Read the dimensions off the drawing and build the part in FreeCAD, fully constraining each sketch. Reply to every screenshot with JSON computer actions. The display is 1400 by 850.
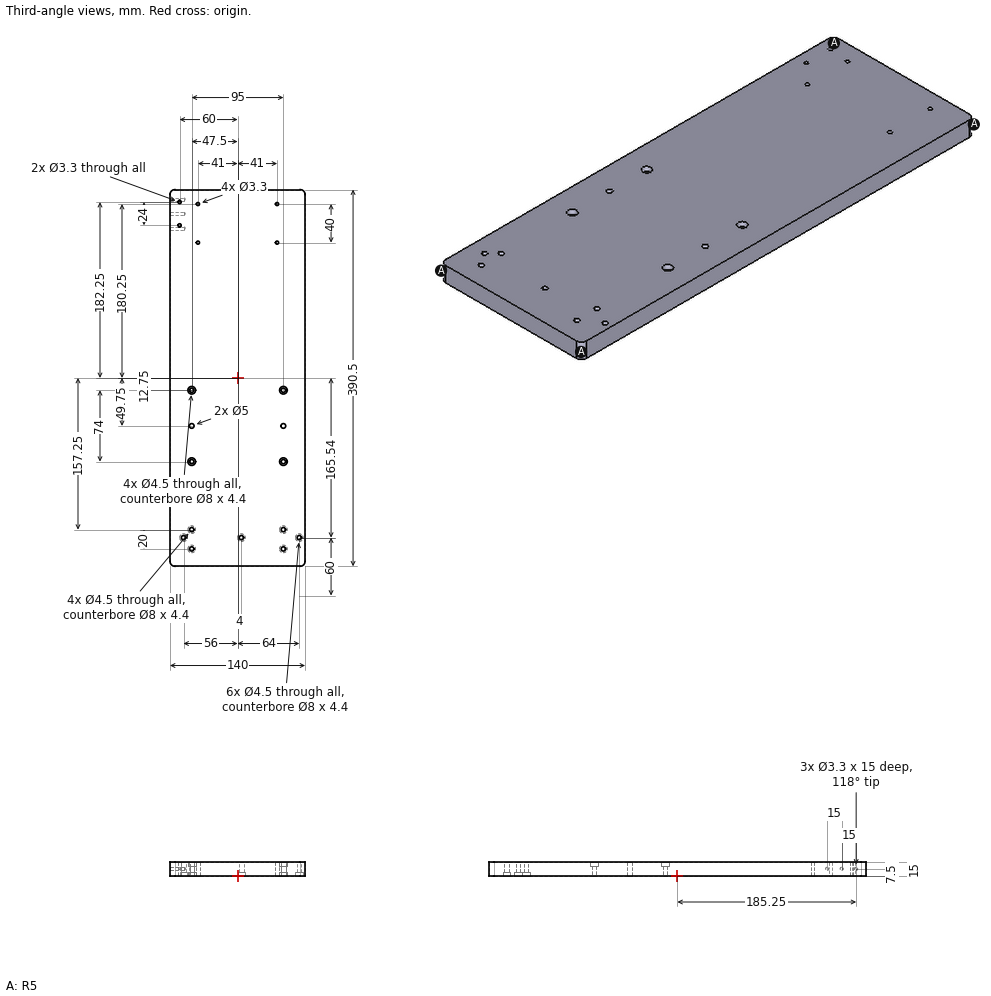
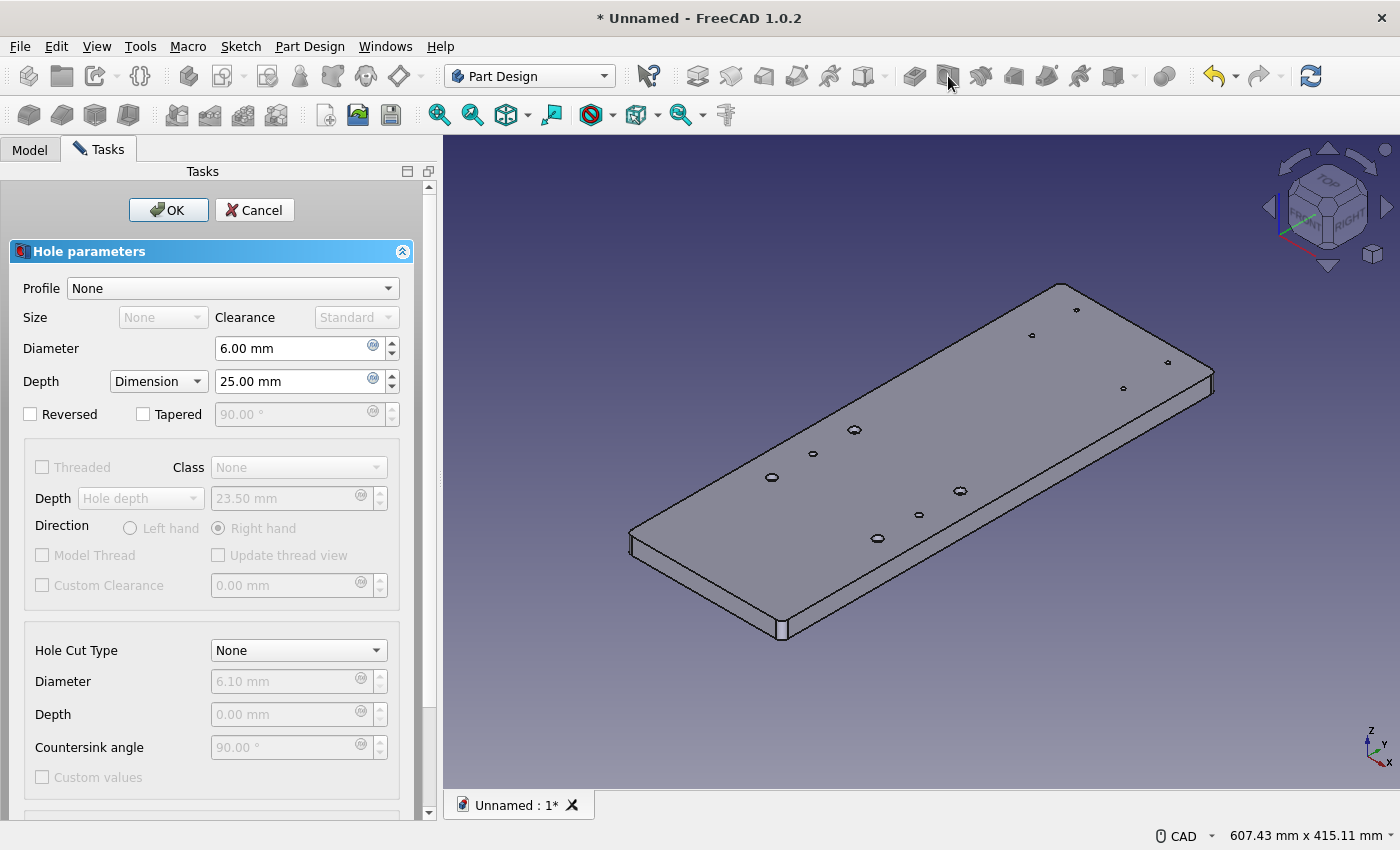
{"action": "triple_click", "coordinate": [300, 348]}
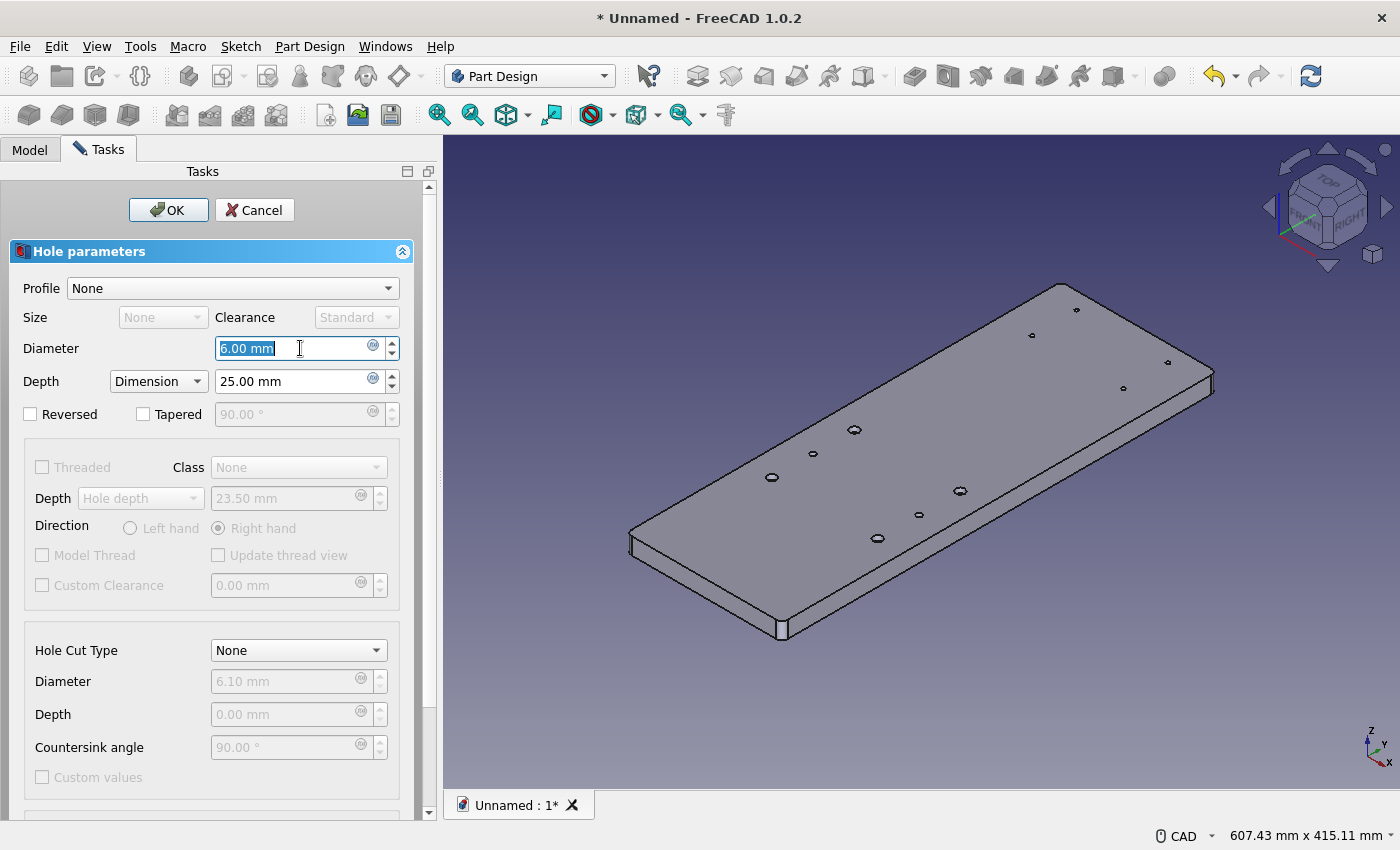
{"action": "type", "text": "4.5"}
{"action": "key", "text": "Tab"}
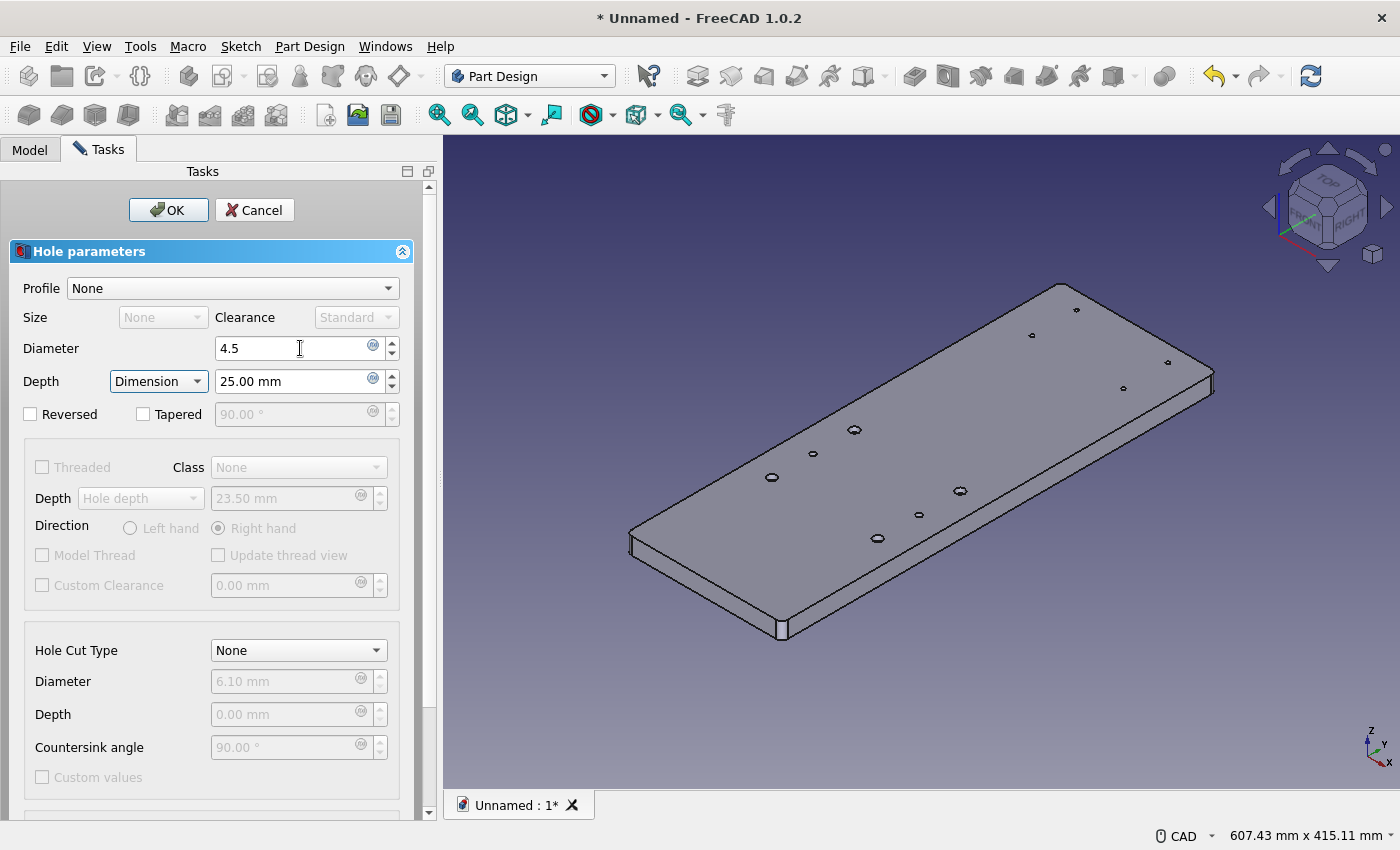
{"action": "left_click", "coordinate": [160, 382]}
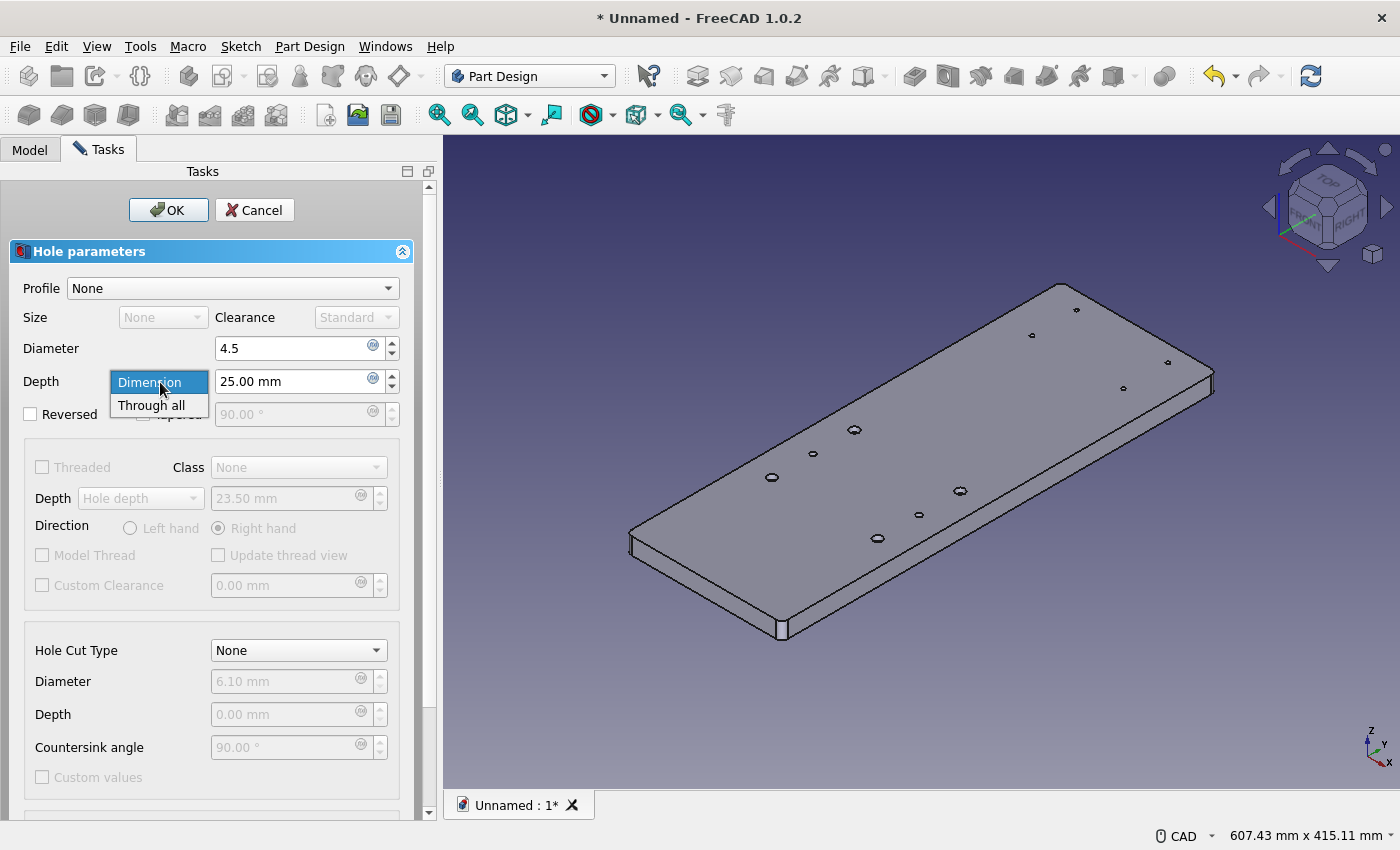
{"action": "left_click", "coordinate": [158, 406]}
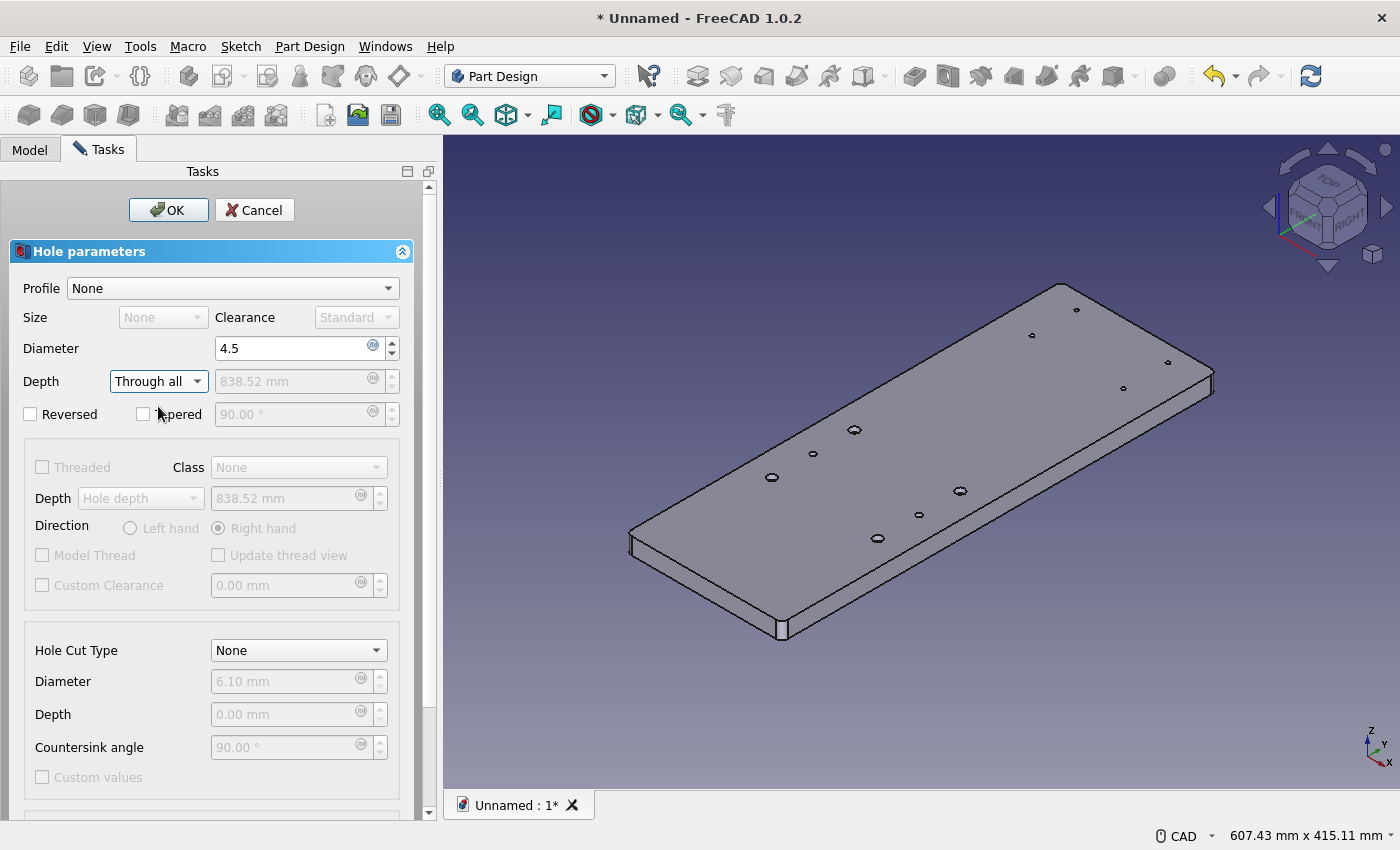
{"action": "left_click", "coordinate": [31, 414]}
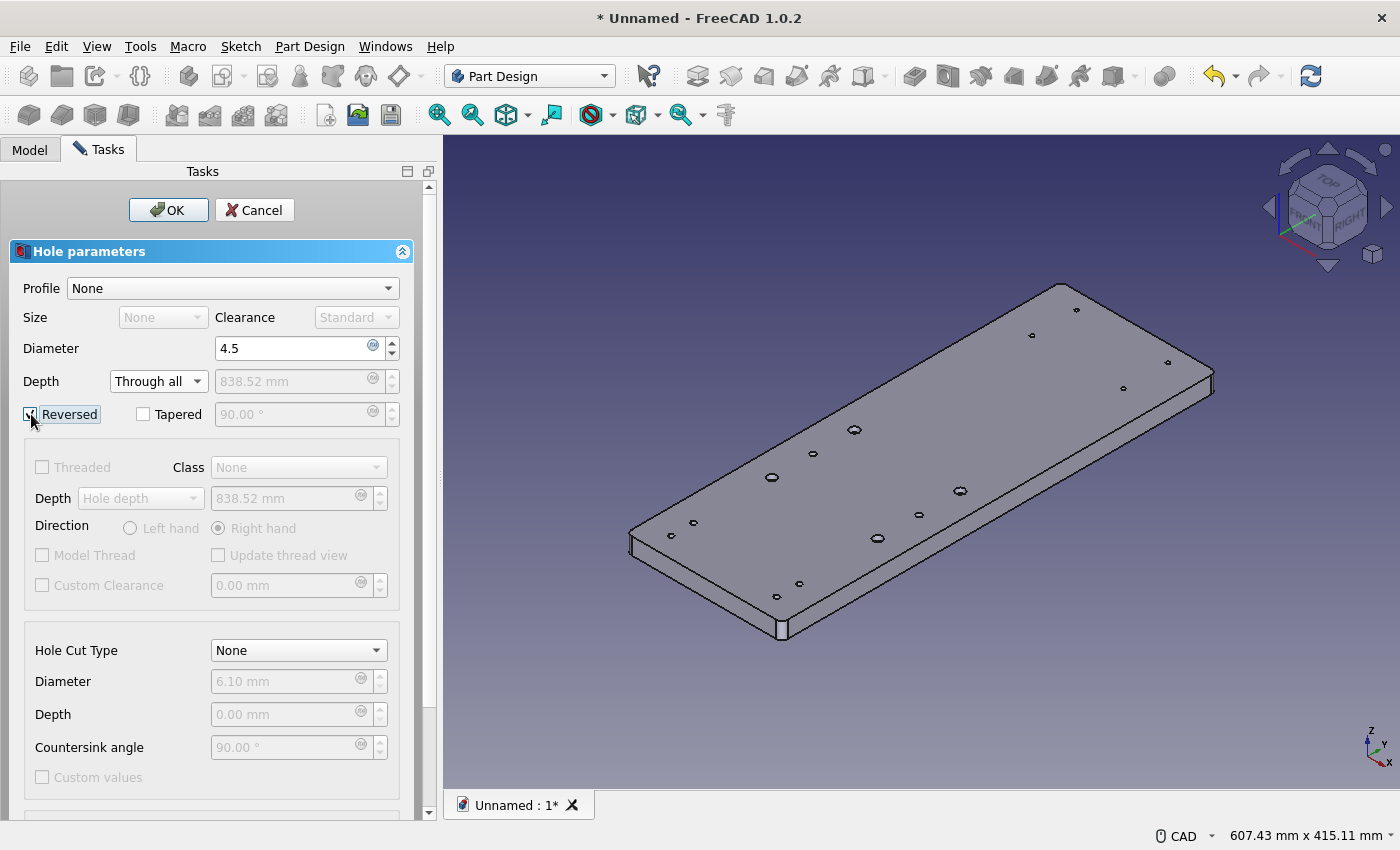
{"action": "left_click", "coordinate": [300, 650]}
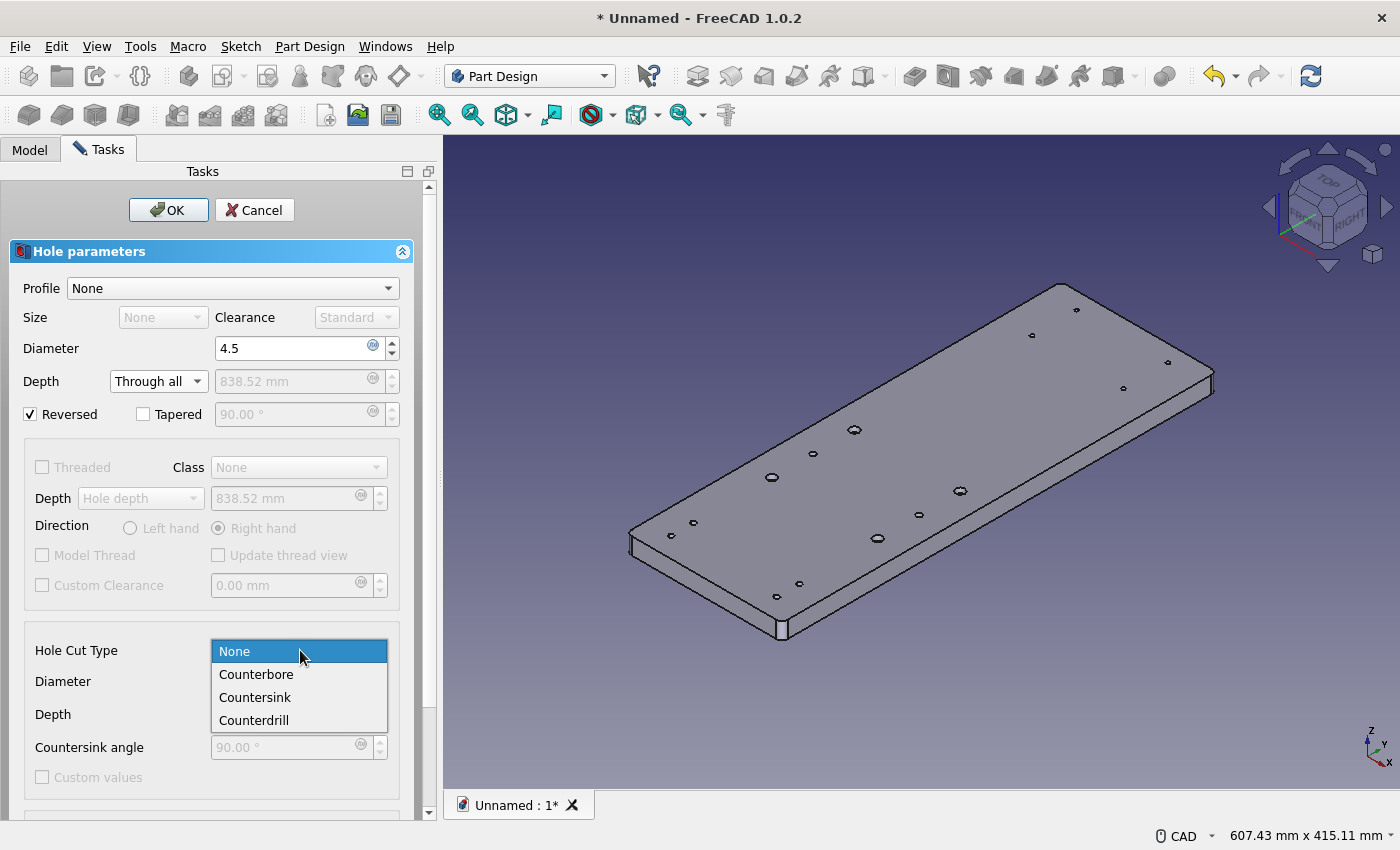
{"action": "left_click", "coordinate": [298, 674]}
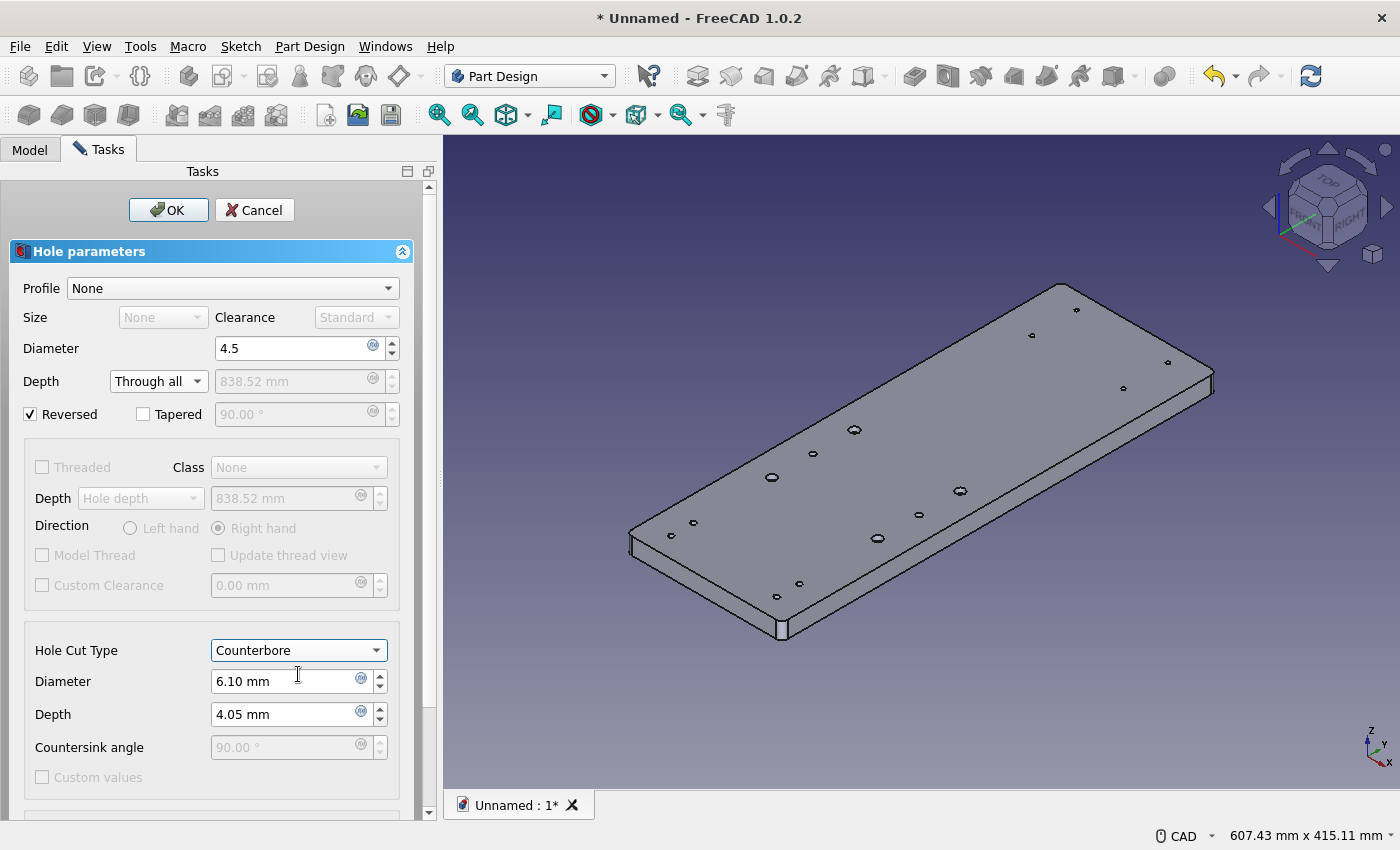
{"action": "triple_click", "coordinate": [292, 682]}